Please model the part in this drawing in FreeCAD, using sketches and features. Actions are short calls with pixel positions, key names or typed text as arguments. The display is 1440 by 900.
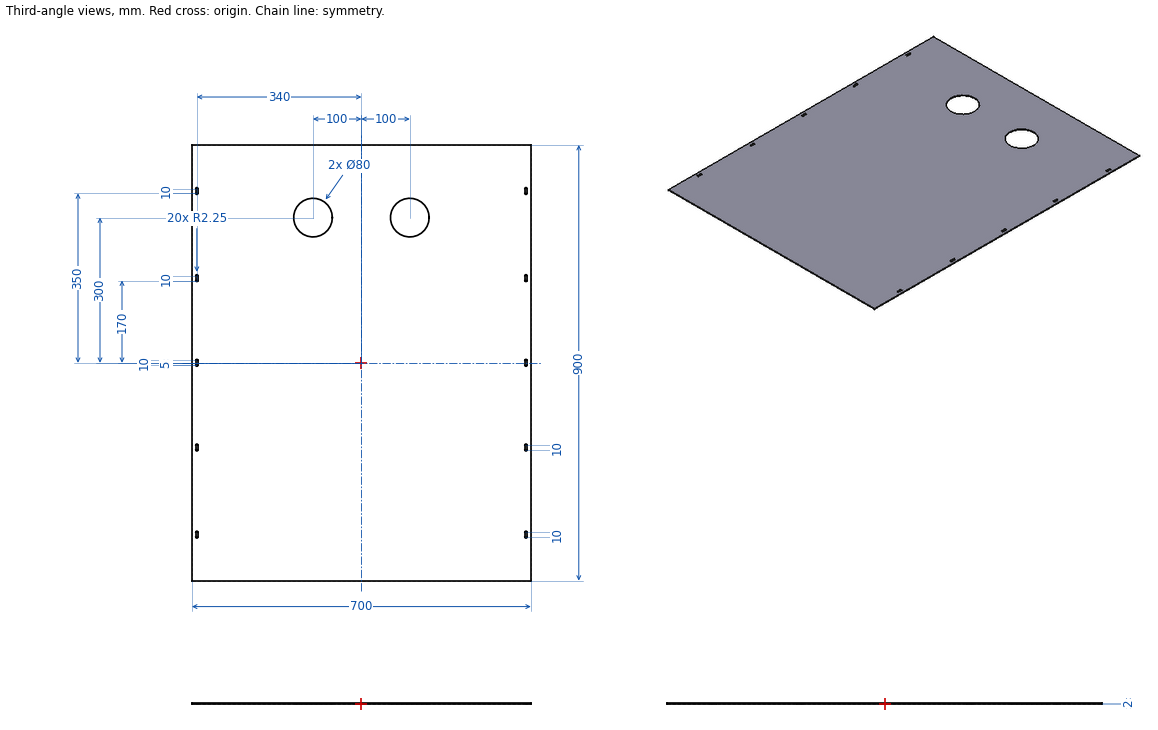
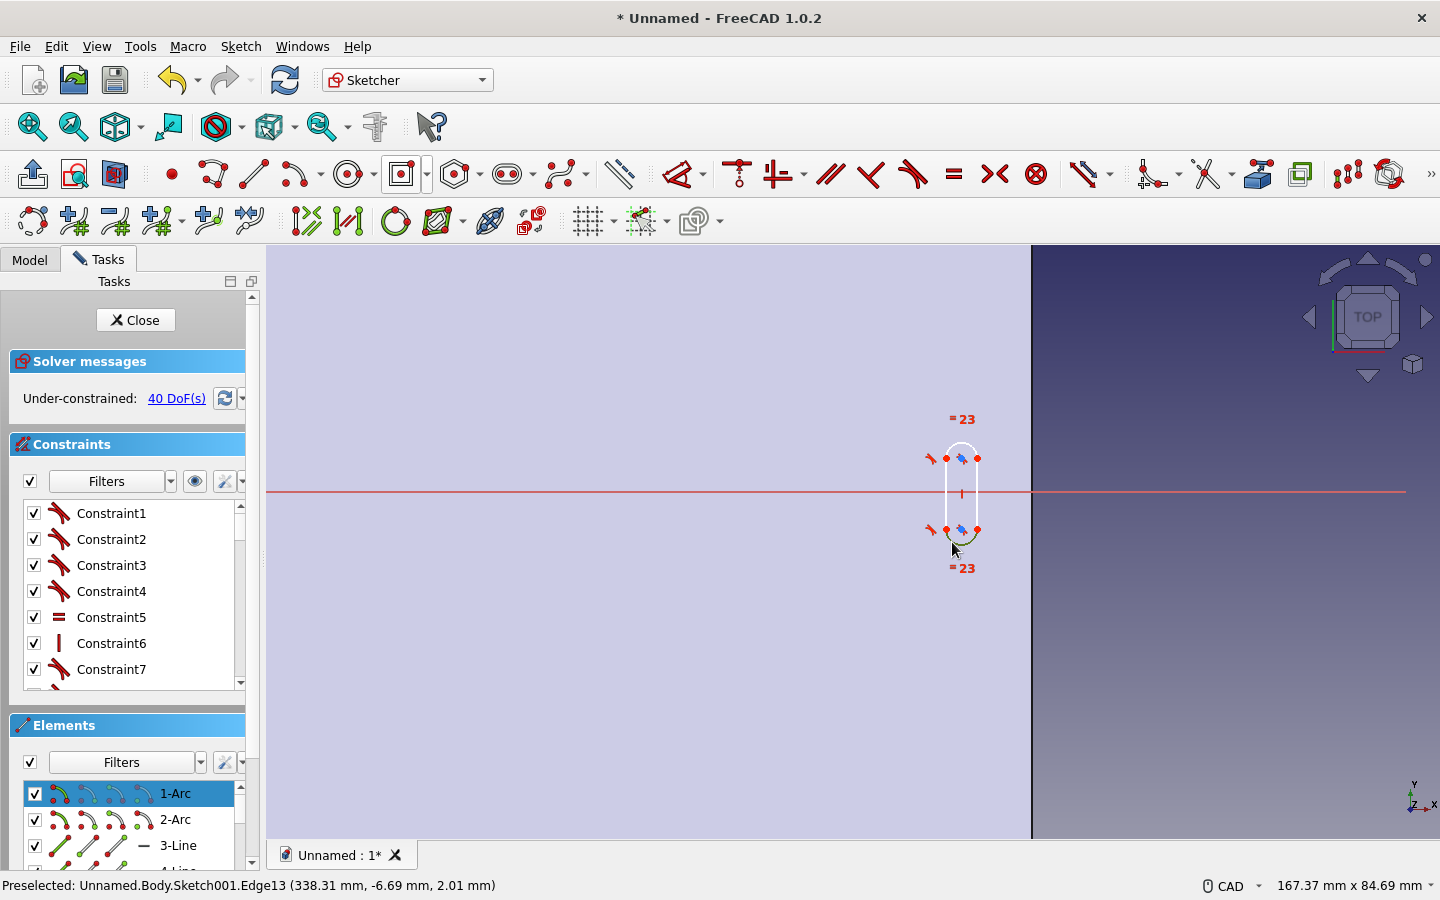
scroll(962, 546, down, 13)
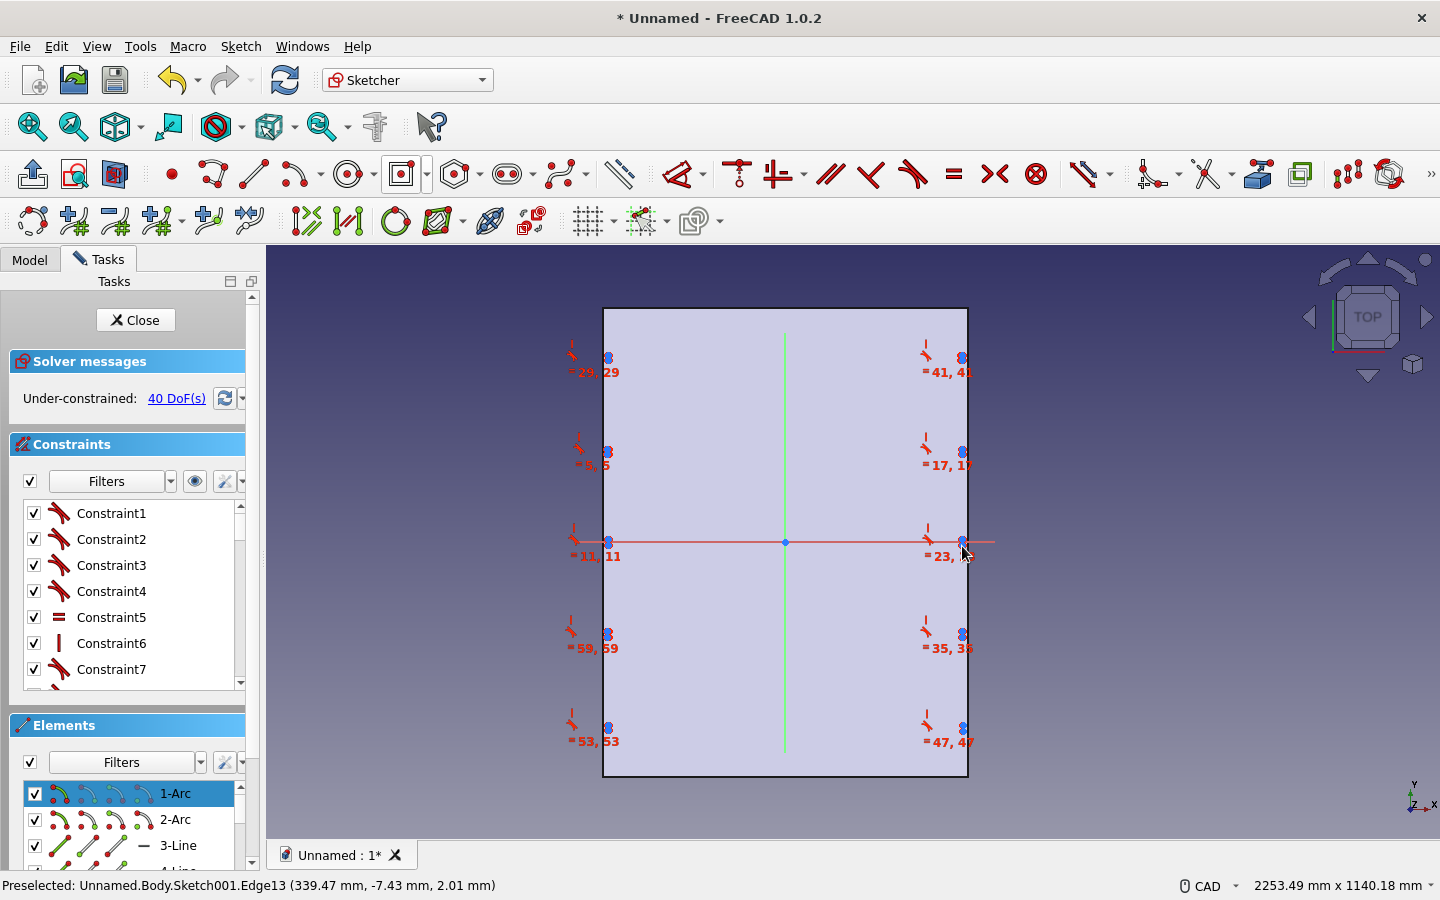
scroll(608, 362, up, 13)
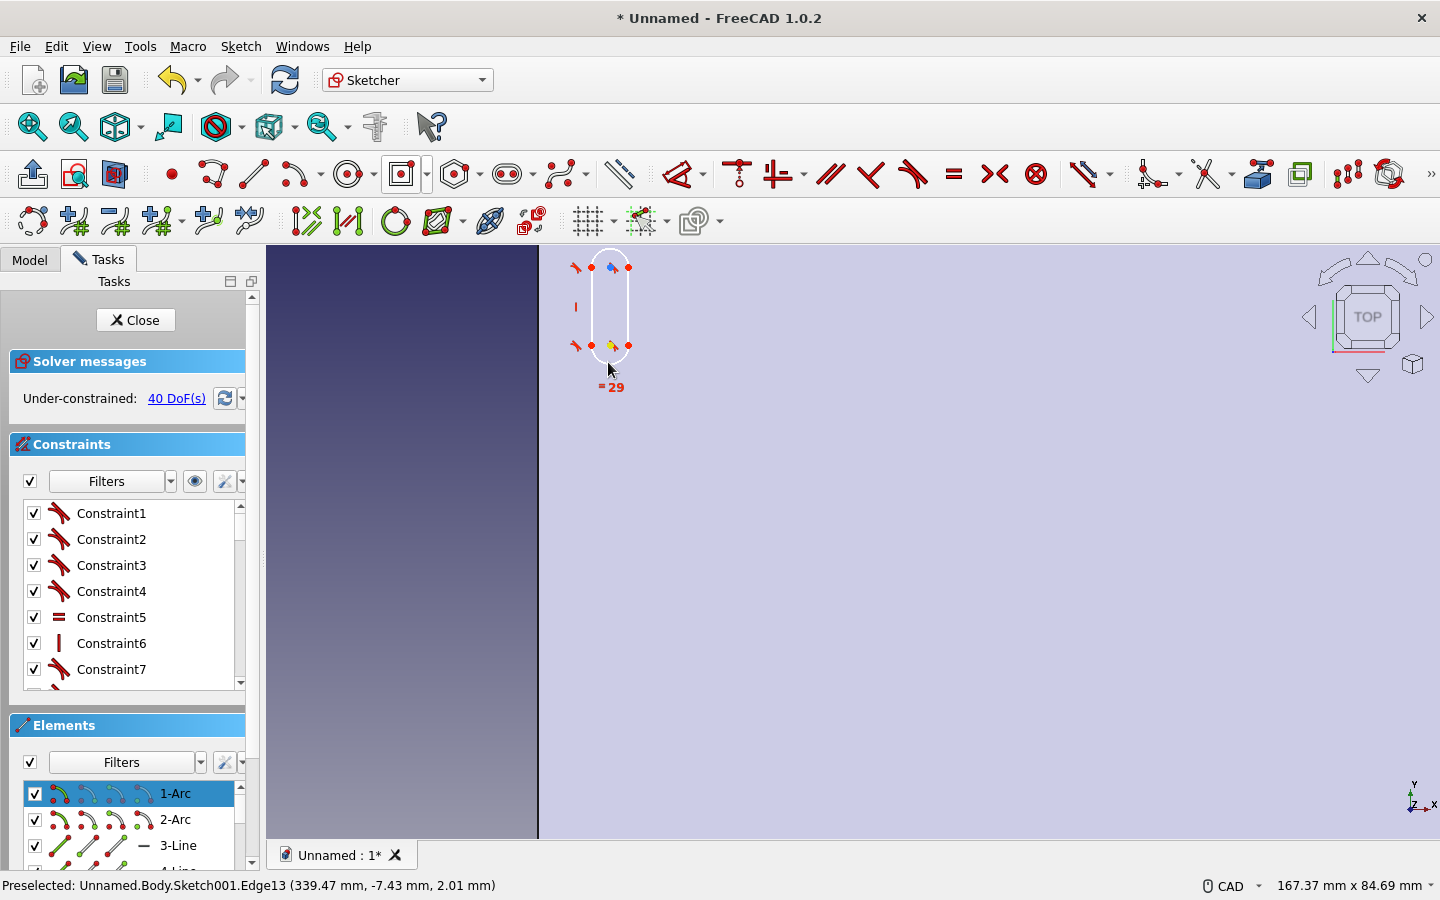
click(599, 361)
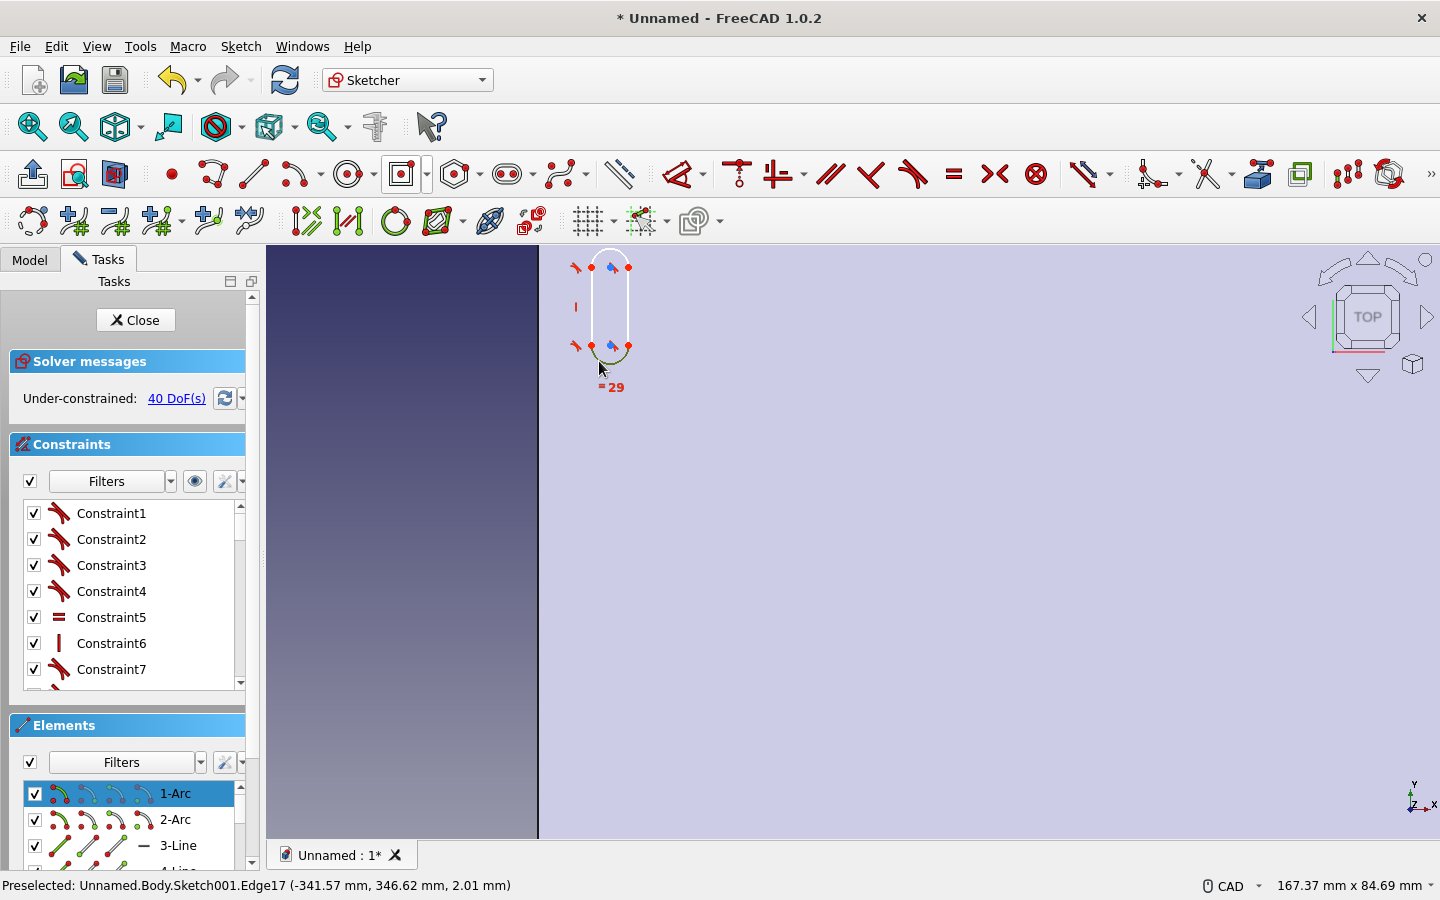
scroll(607, 362, down, 13)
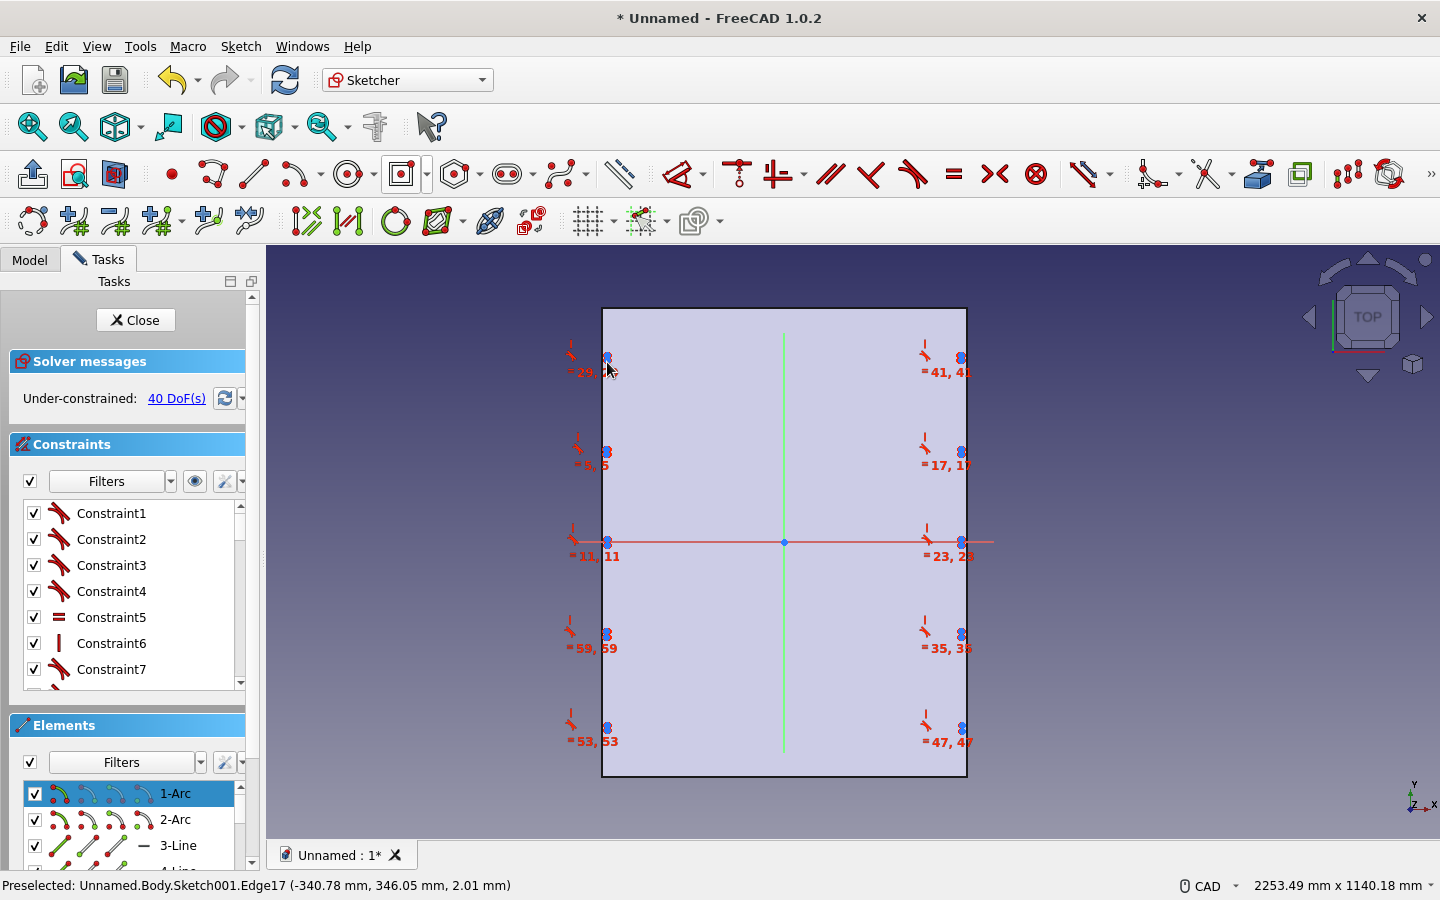
scroll(961, 638, up, 14)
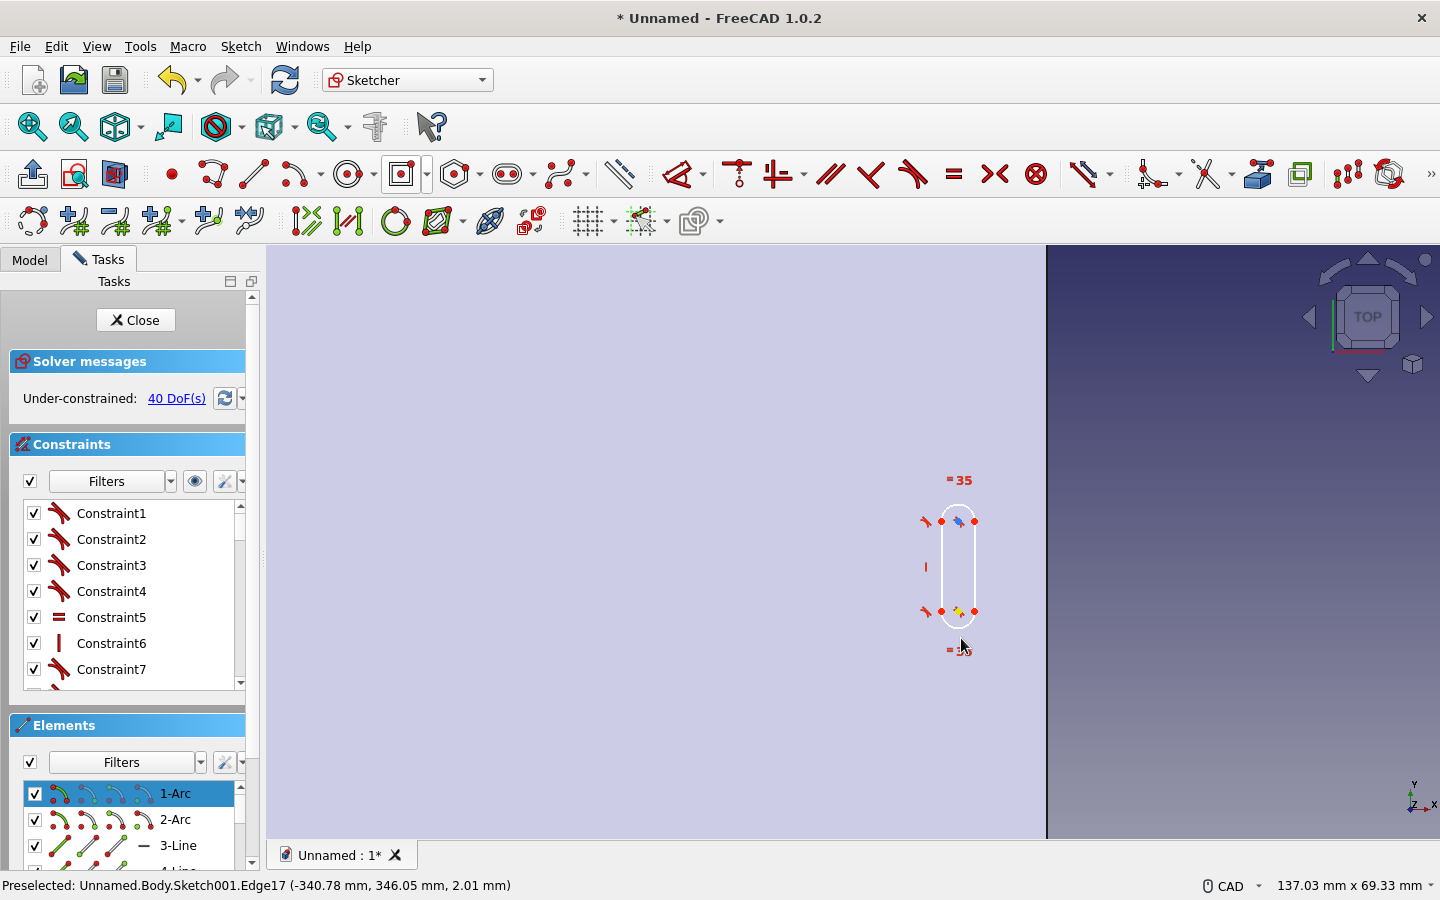
click(948, 625)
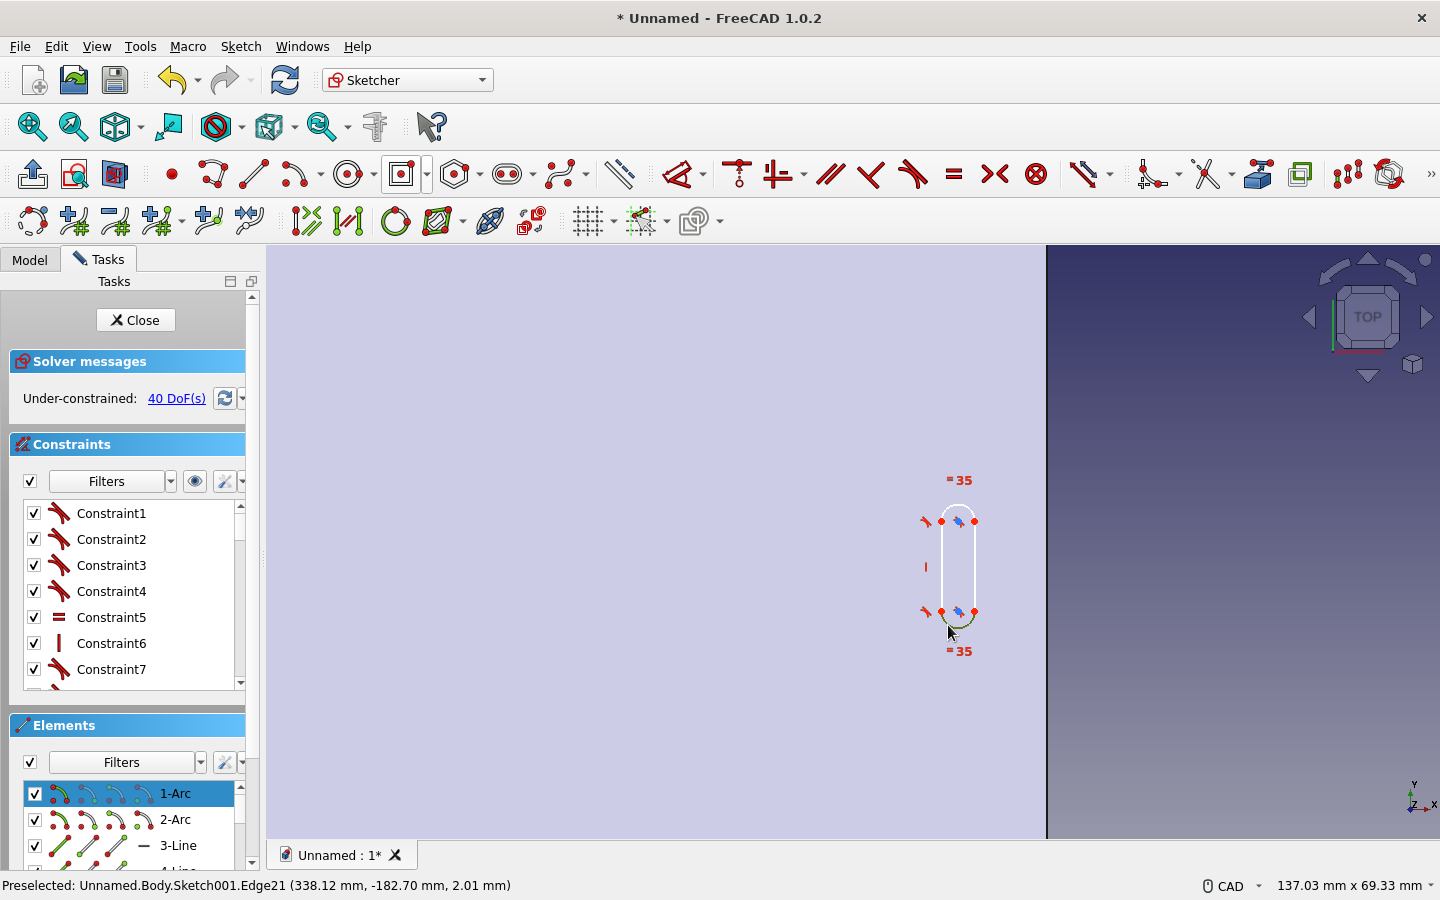
scroll(962, 638, down, 14)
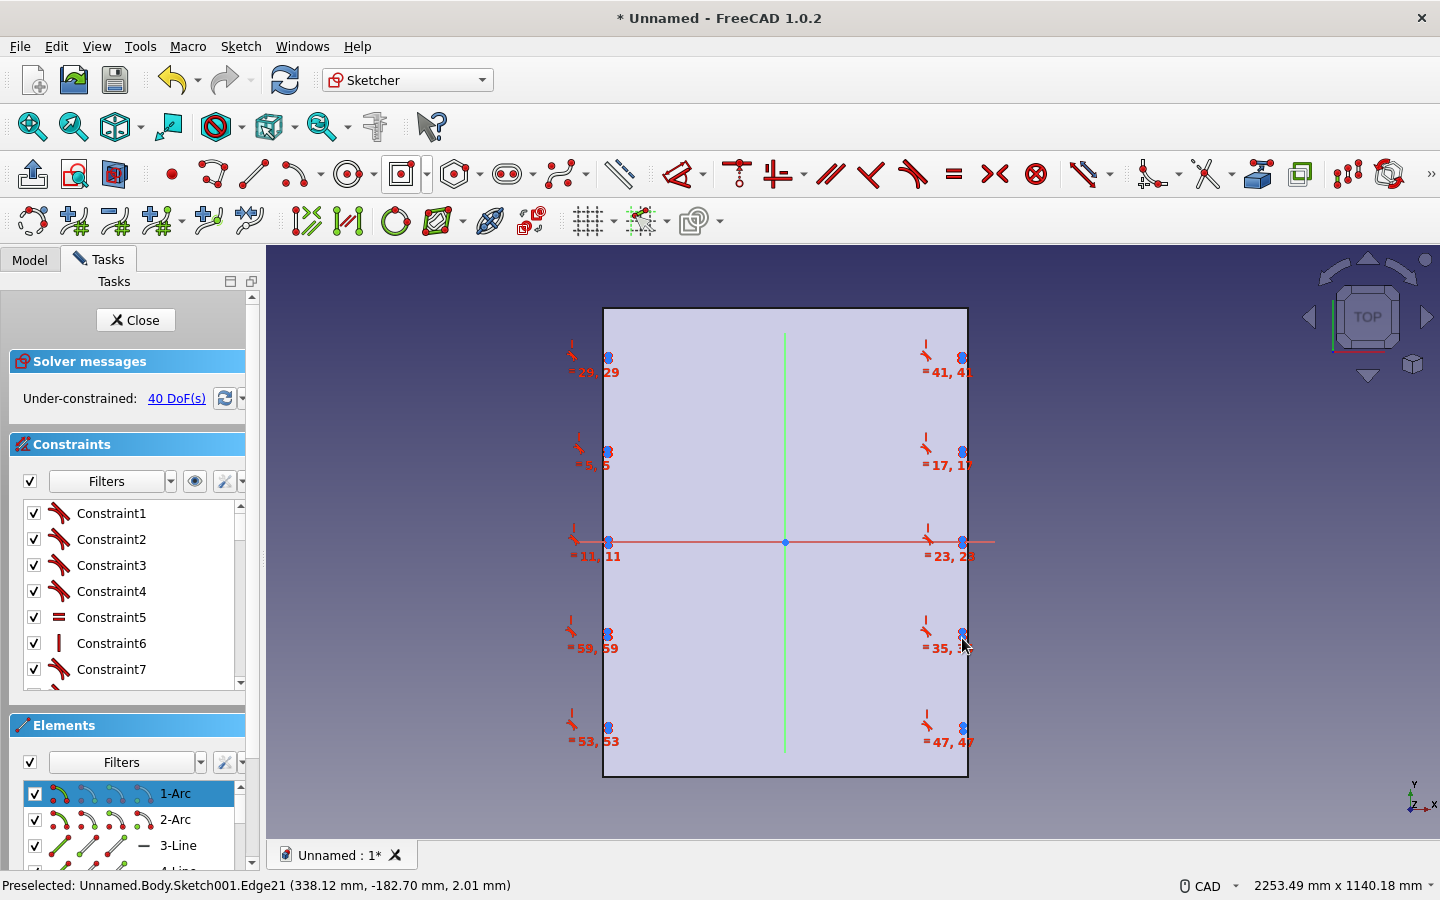
scroll(961, 362, up, 13)